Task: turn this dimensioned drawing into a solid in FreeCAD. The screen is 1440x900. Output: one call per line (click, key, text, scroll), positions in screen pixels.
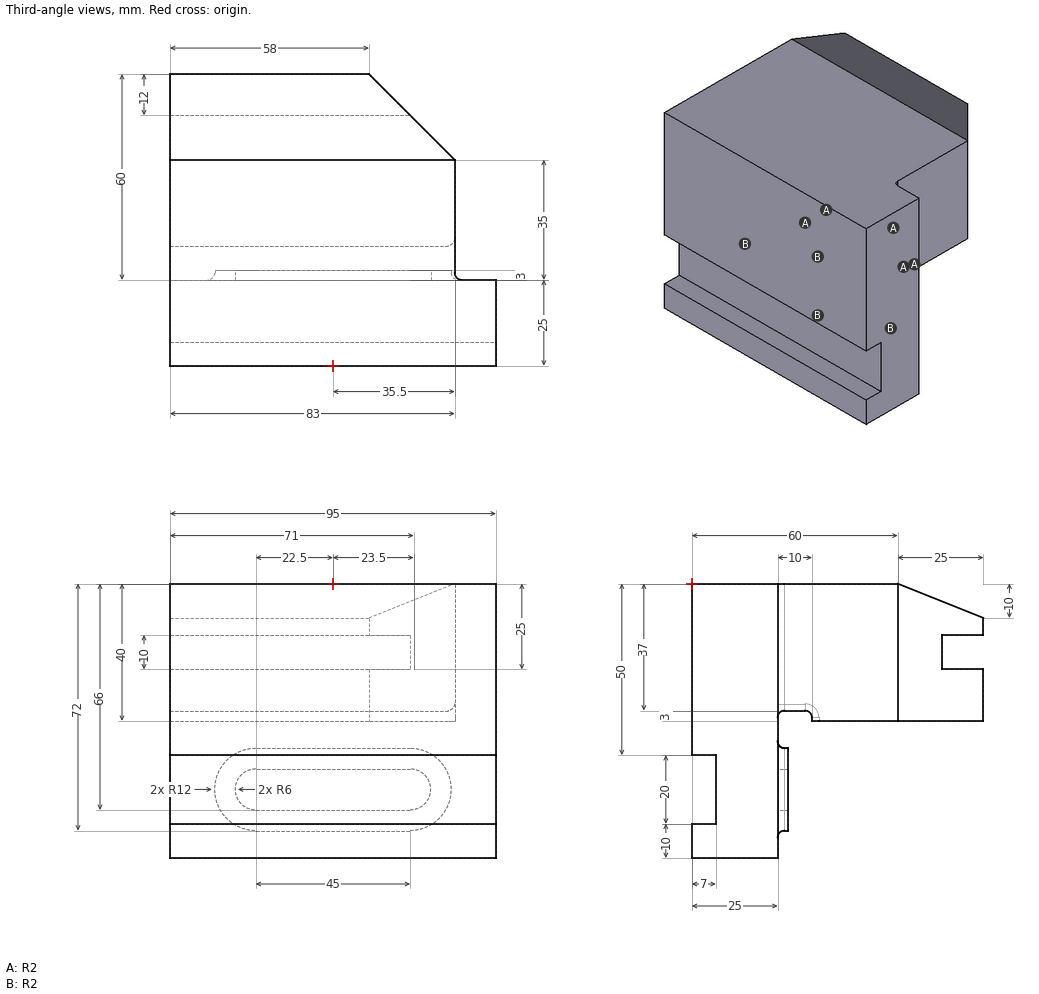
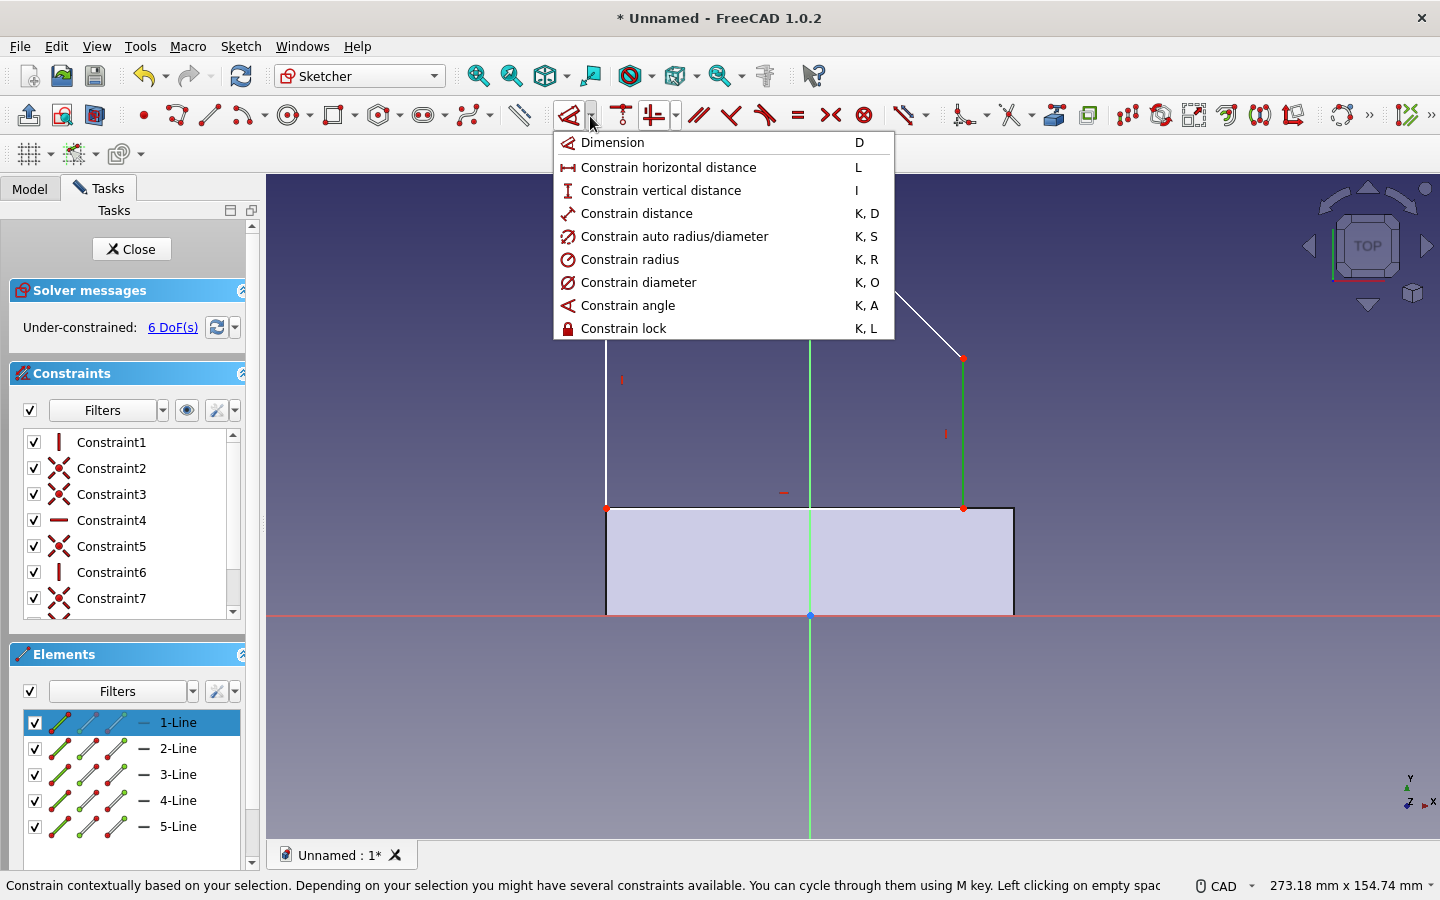
click(724, 190)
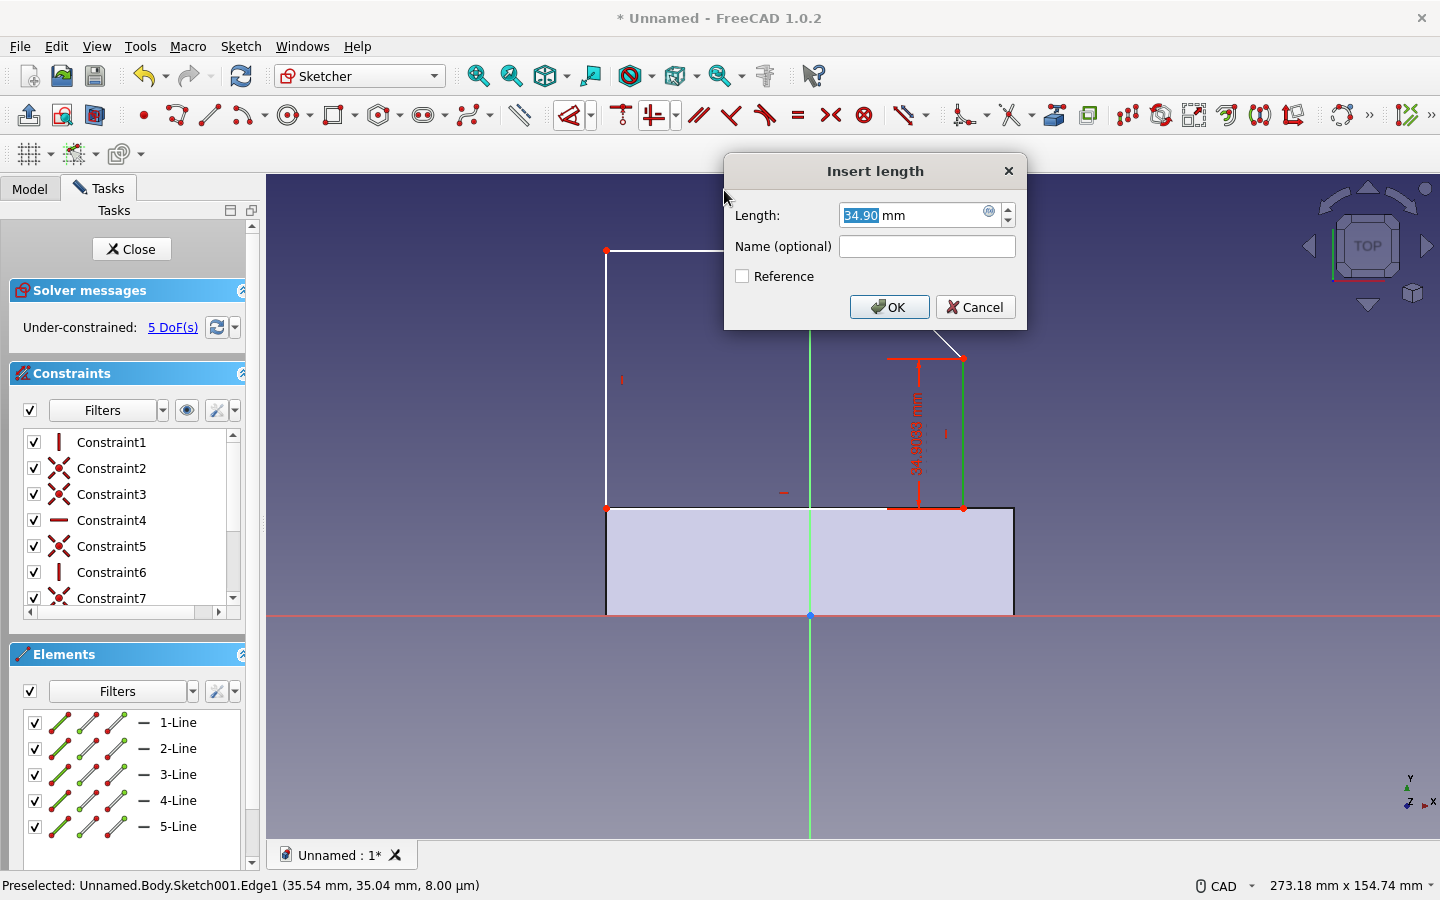
text(35)
key(Return)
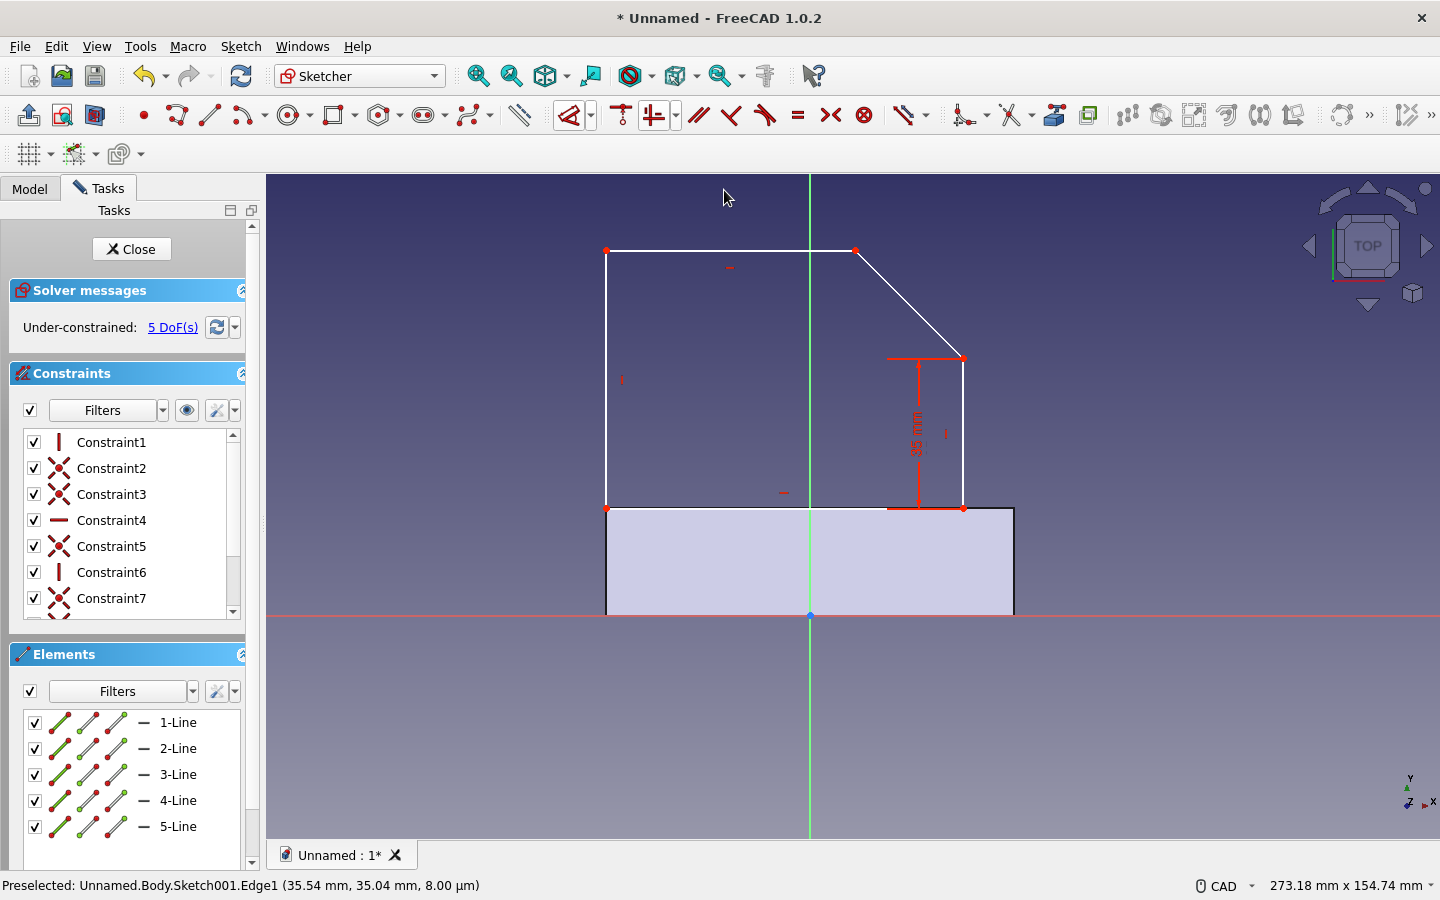
click(780, 251)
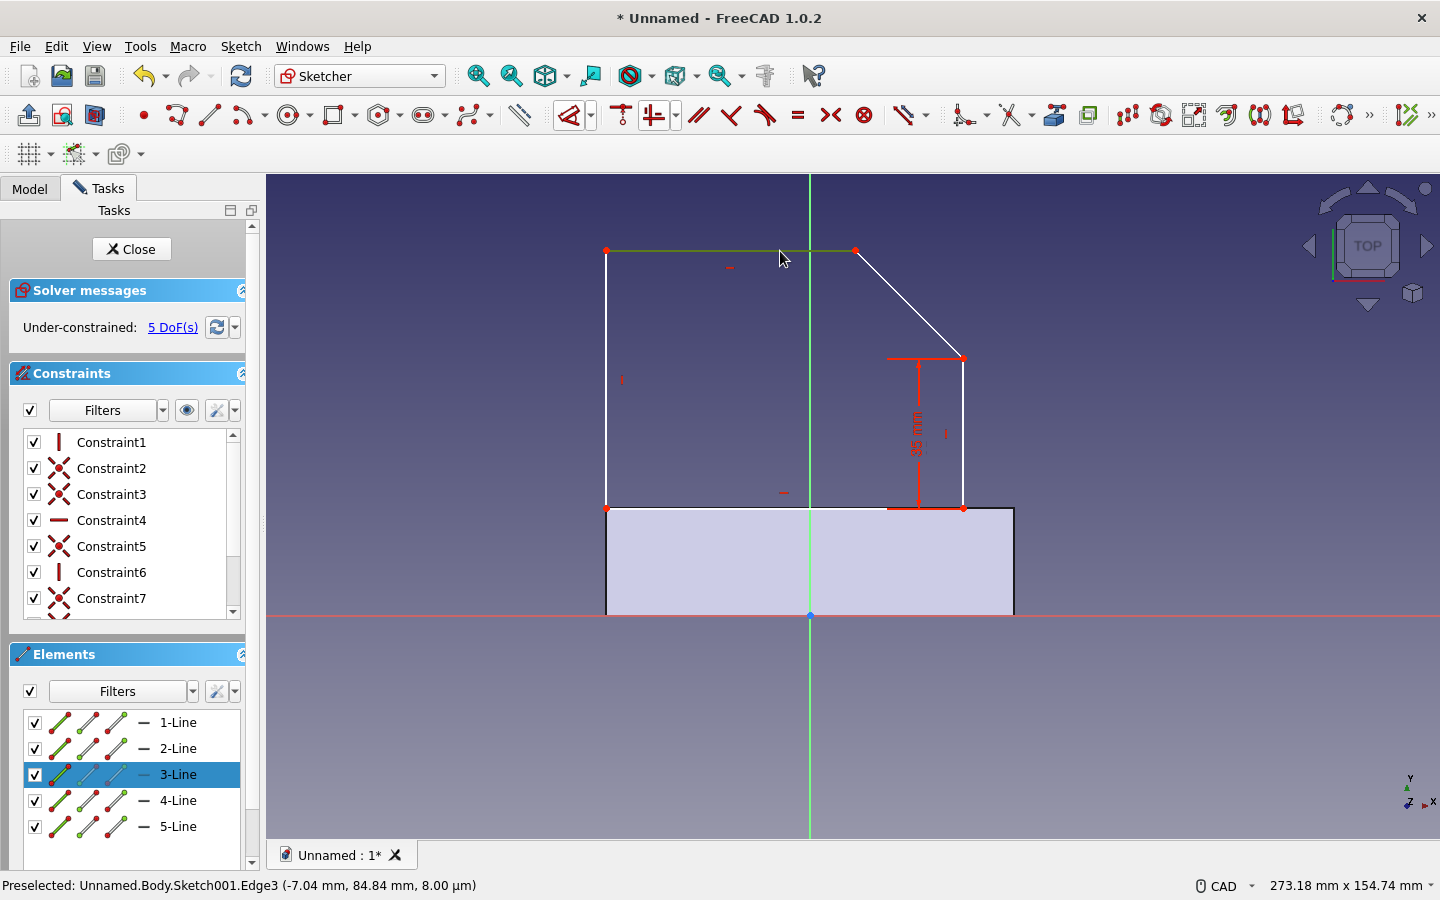
click(590, 116)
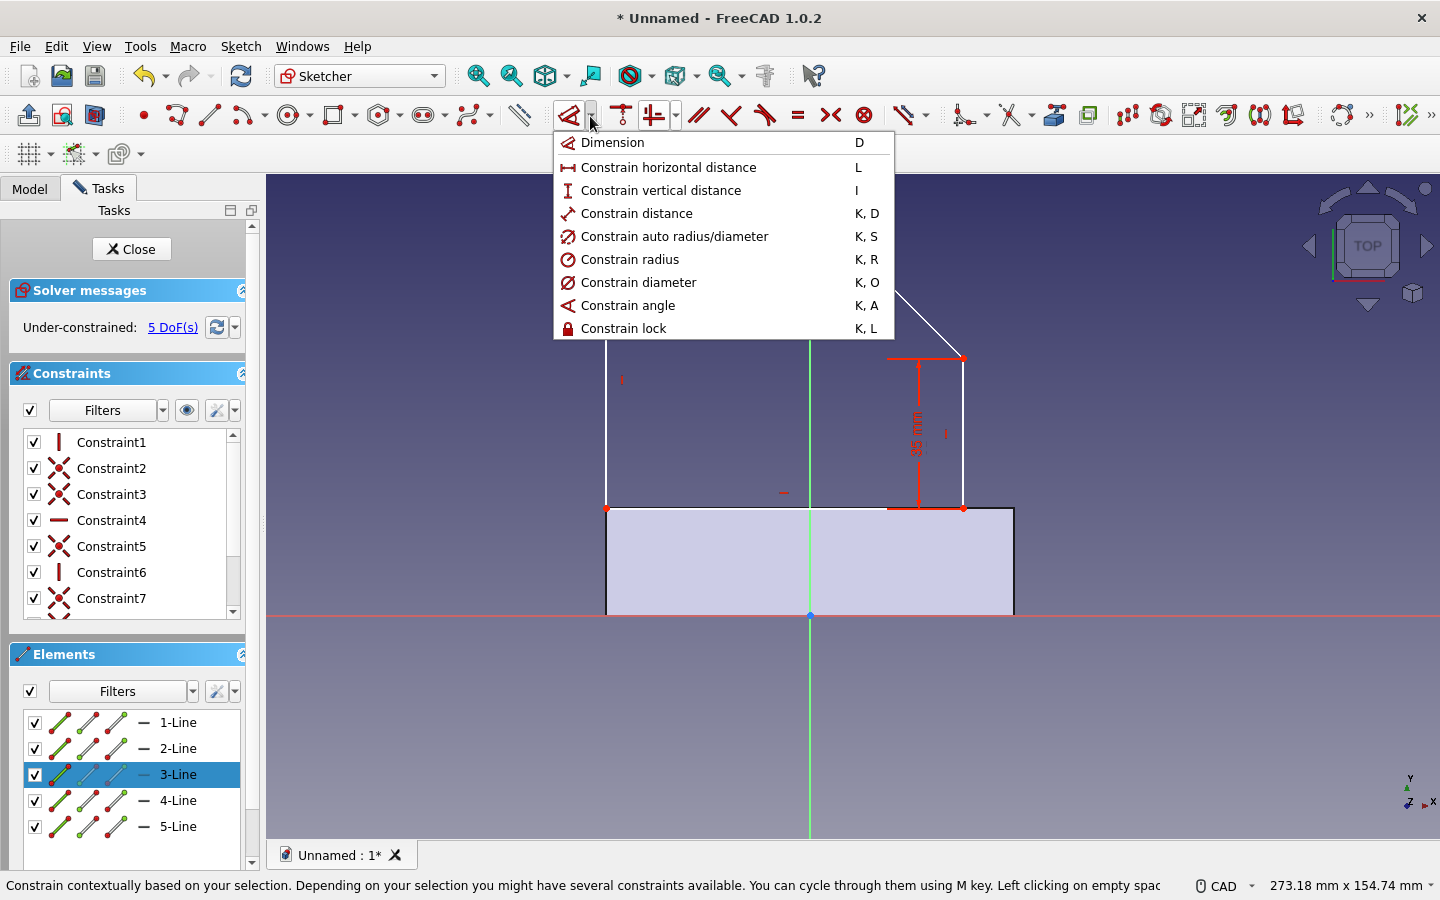
click(724, 168)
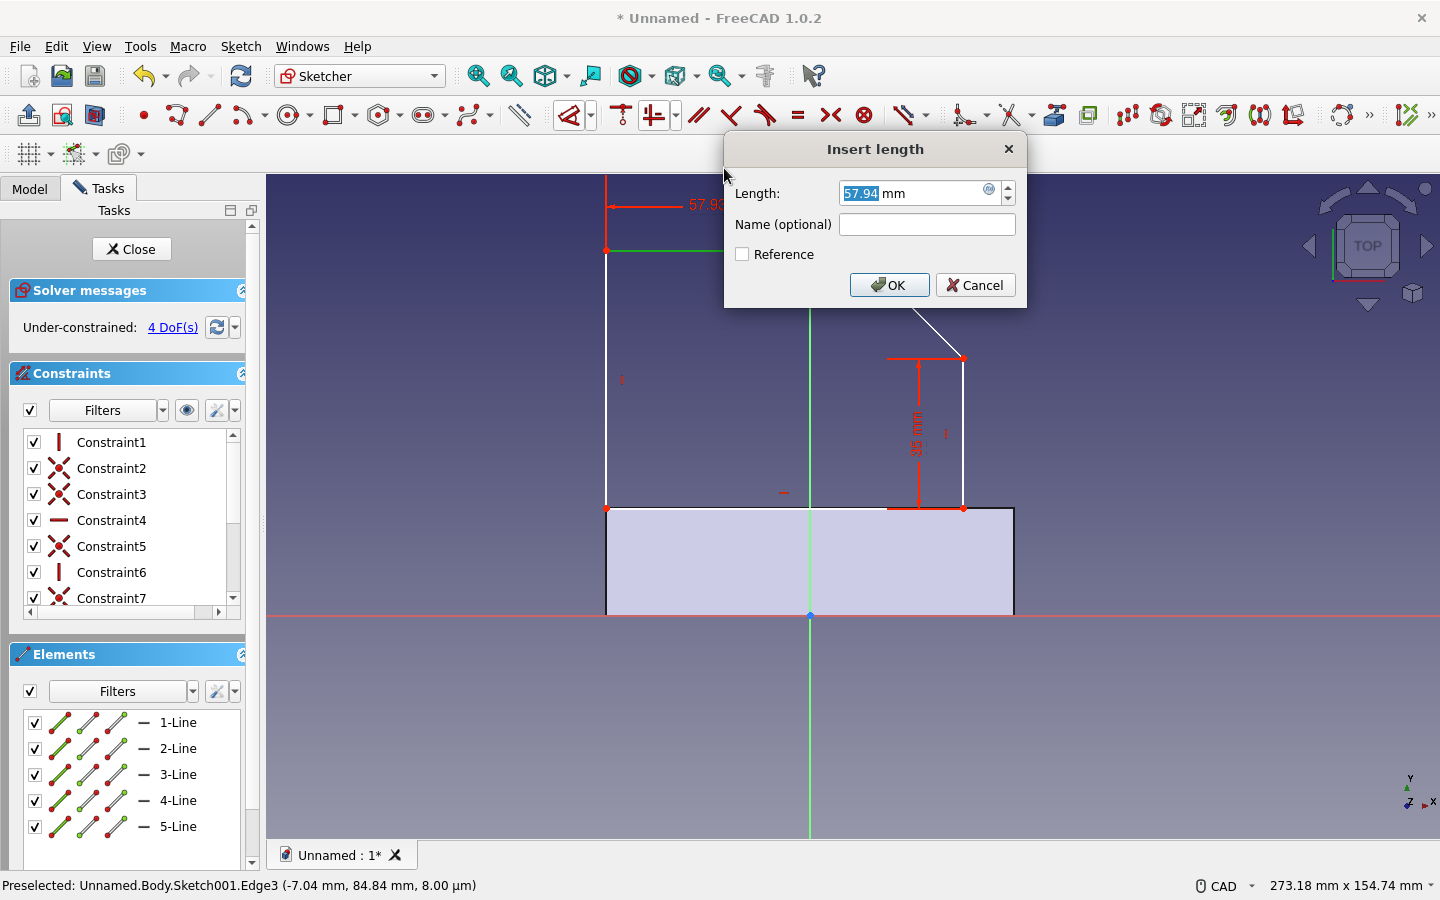
text(58)
key(Return)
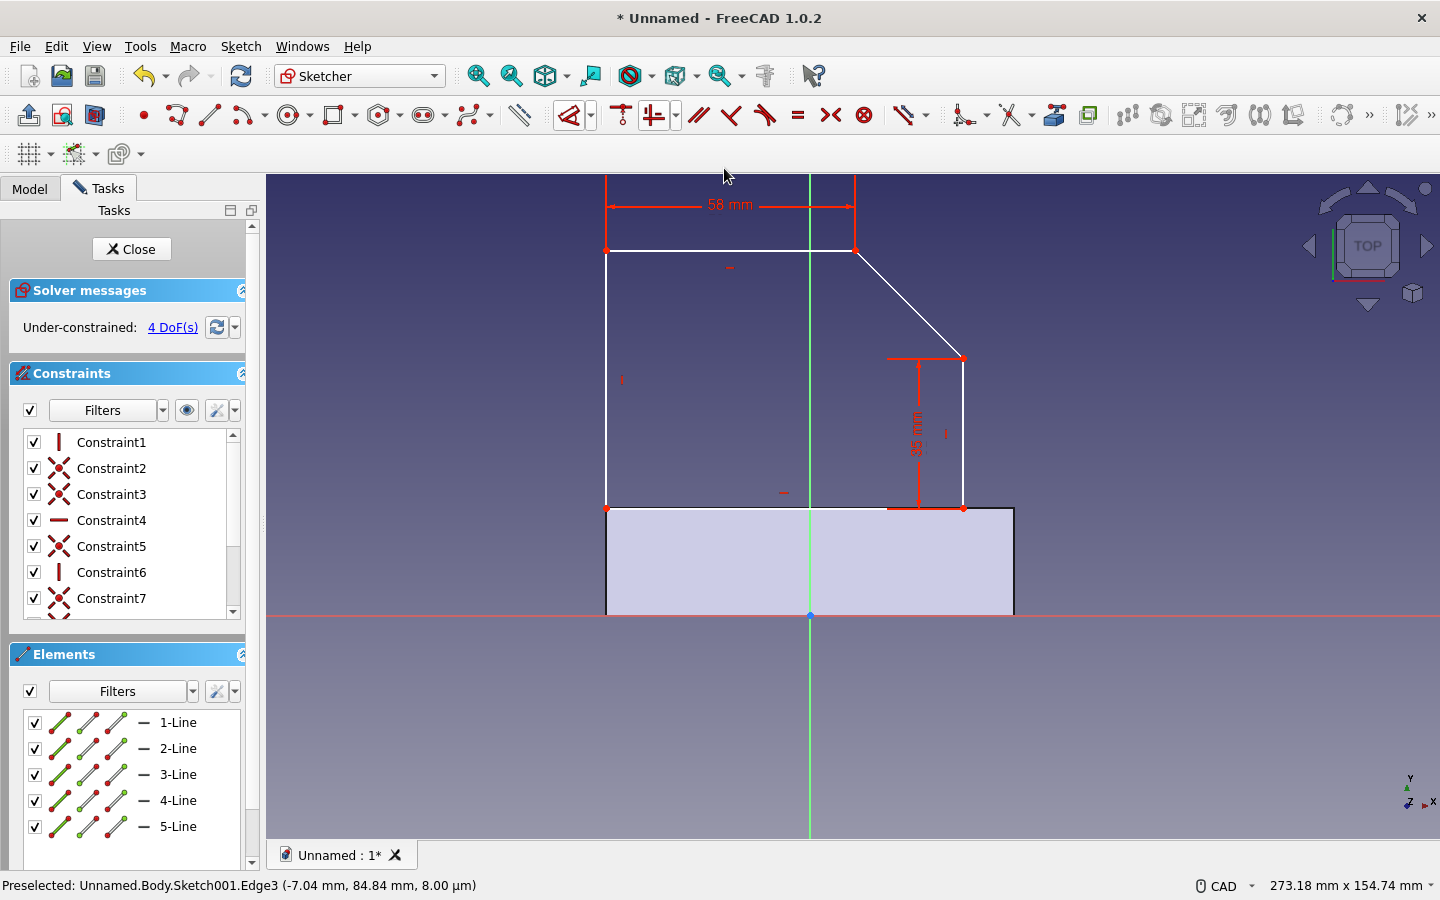
click(606, 328)